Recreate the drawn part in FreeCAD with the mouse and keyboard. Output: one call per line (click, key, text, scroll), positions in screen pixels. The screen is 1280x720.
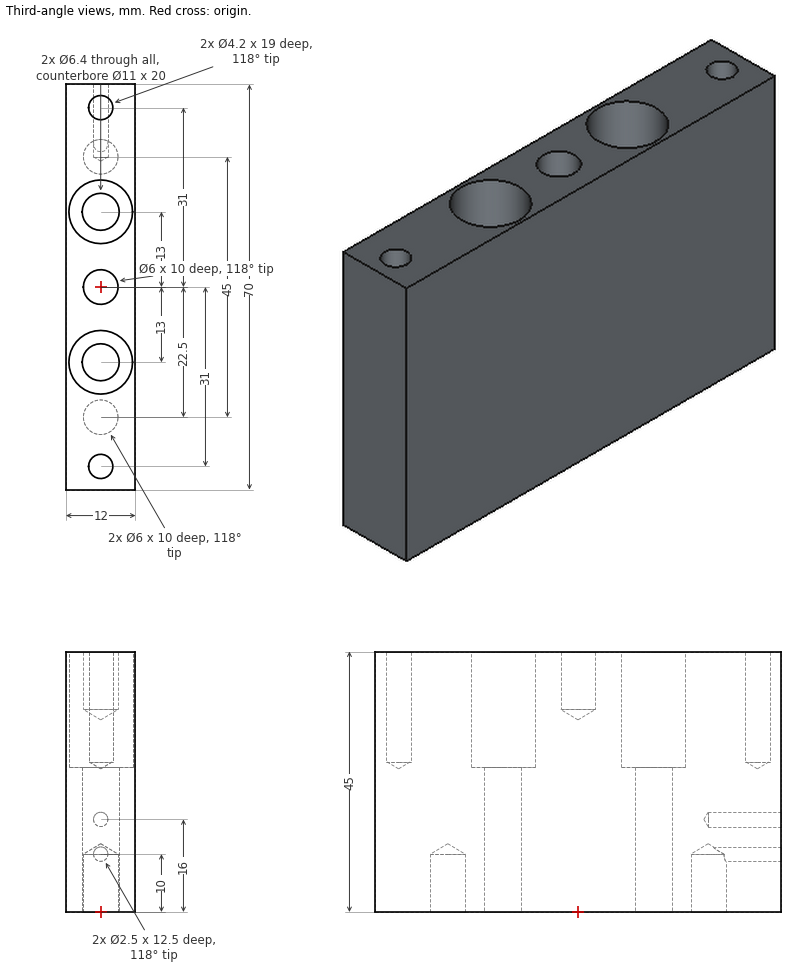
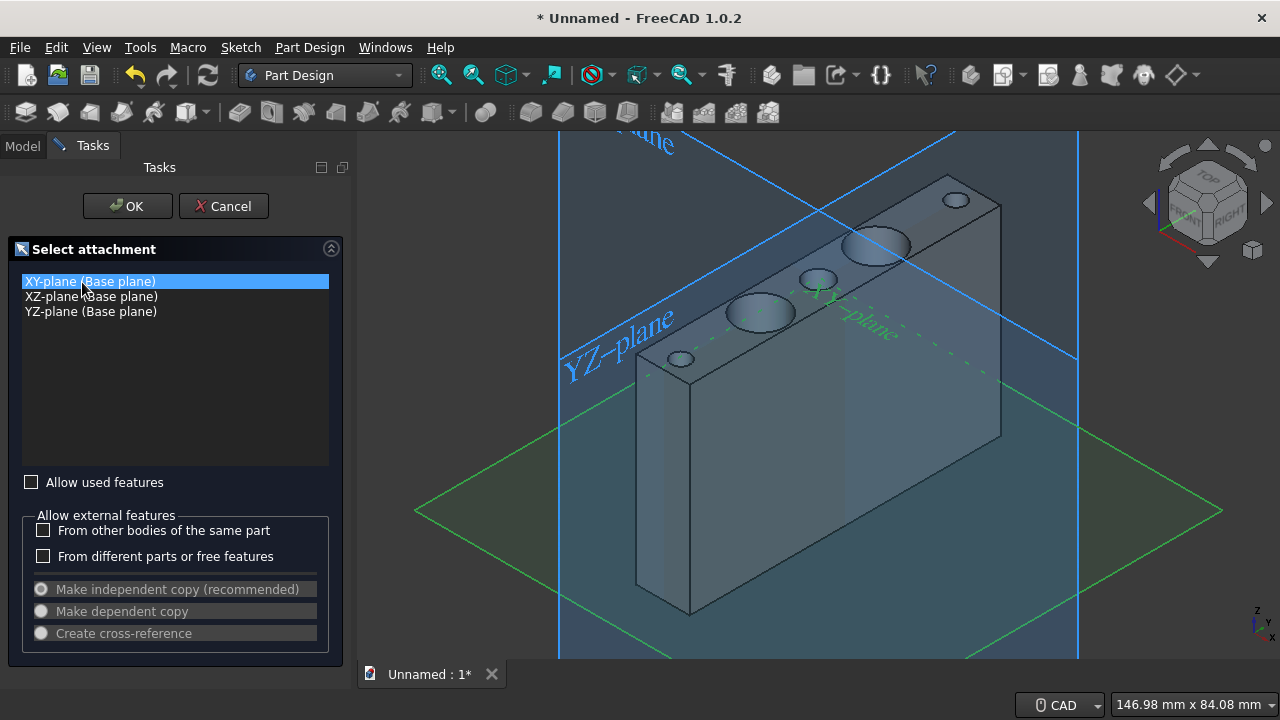
click(128, 206)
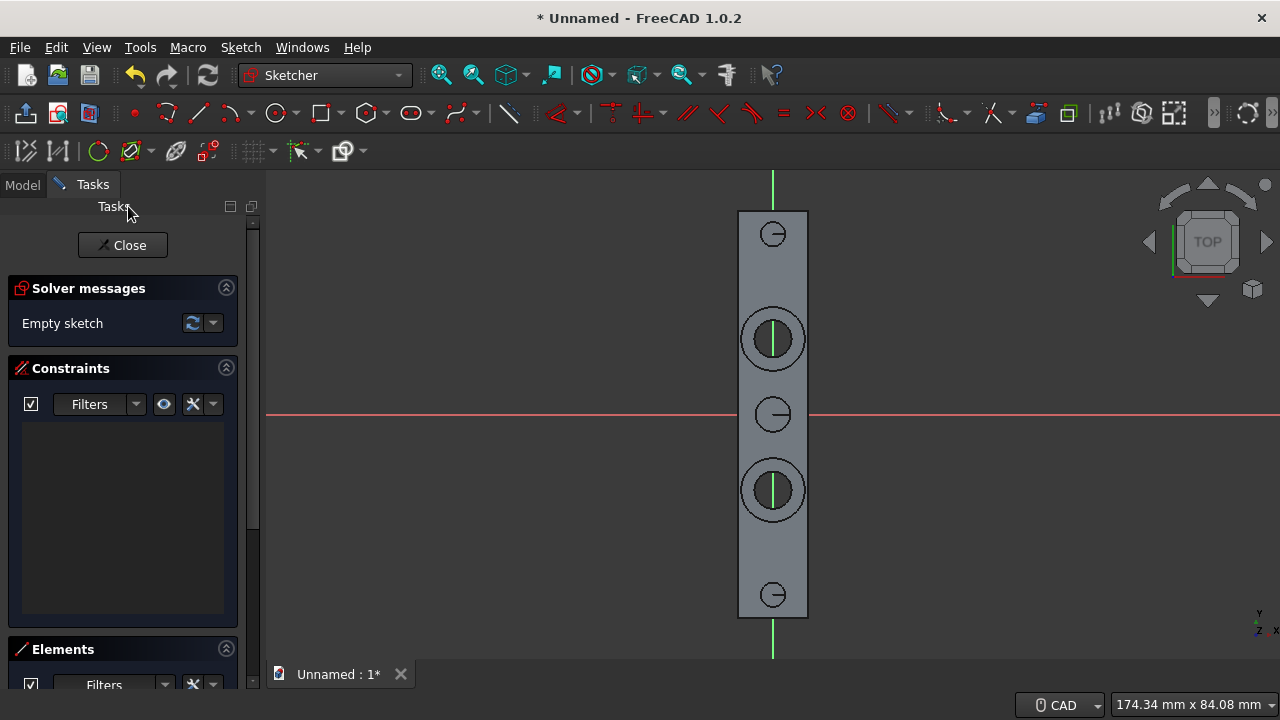
click(90, 114)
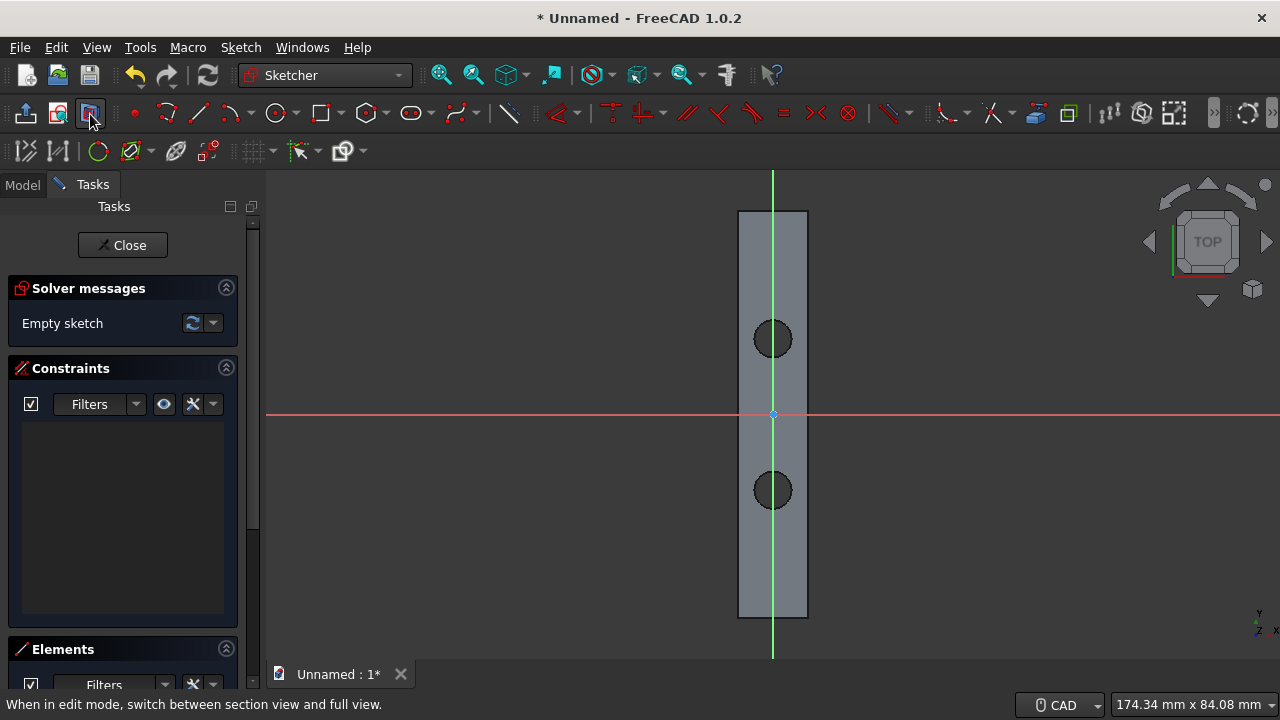
click(276, 114)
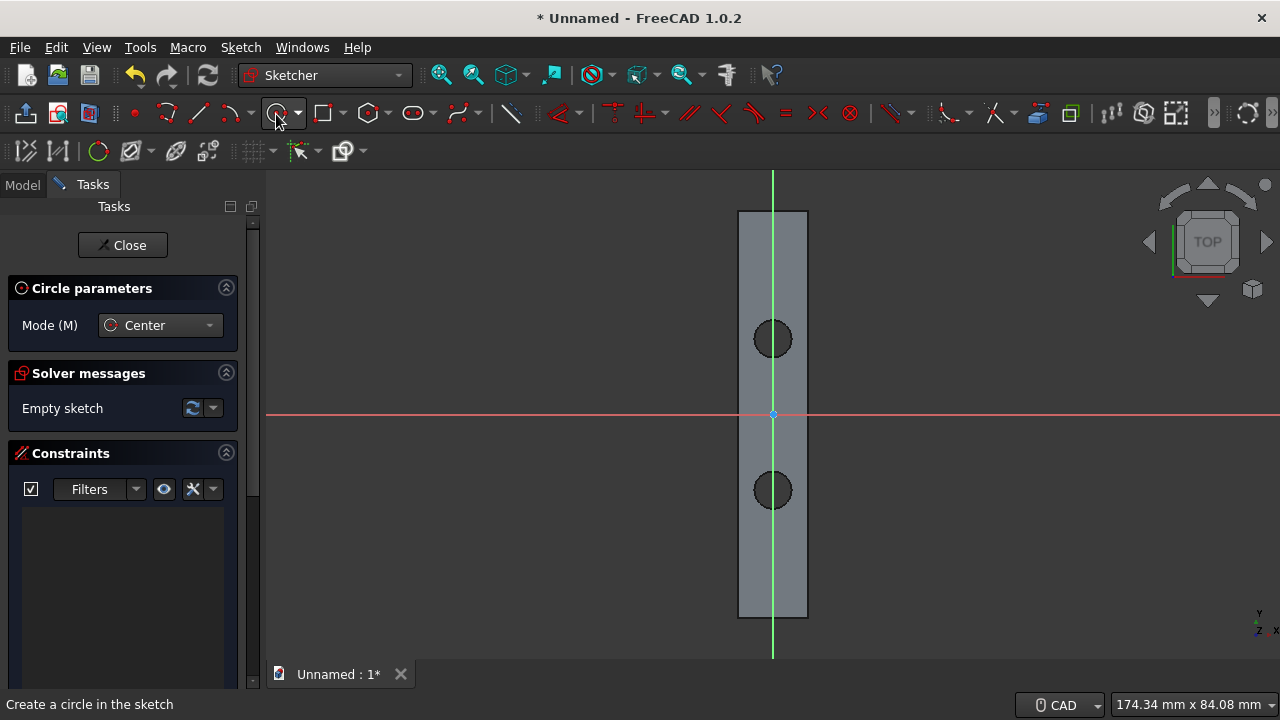
scroll(773, 545, up, 2)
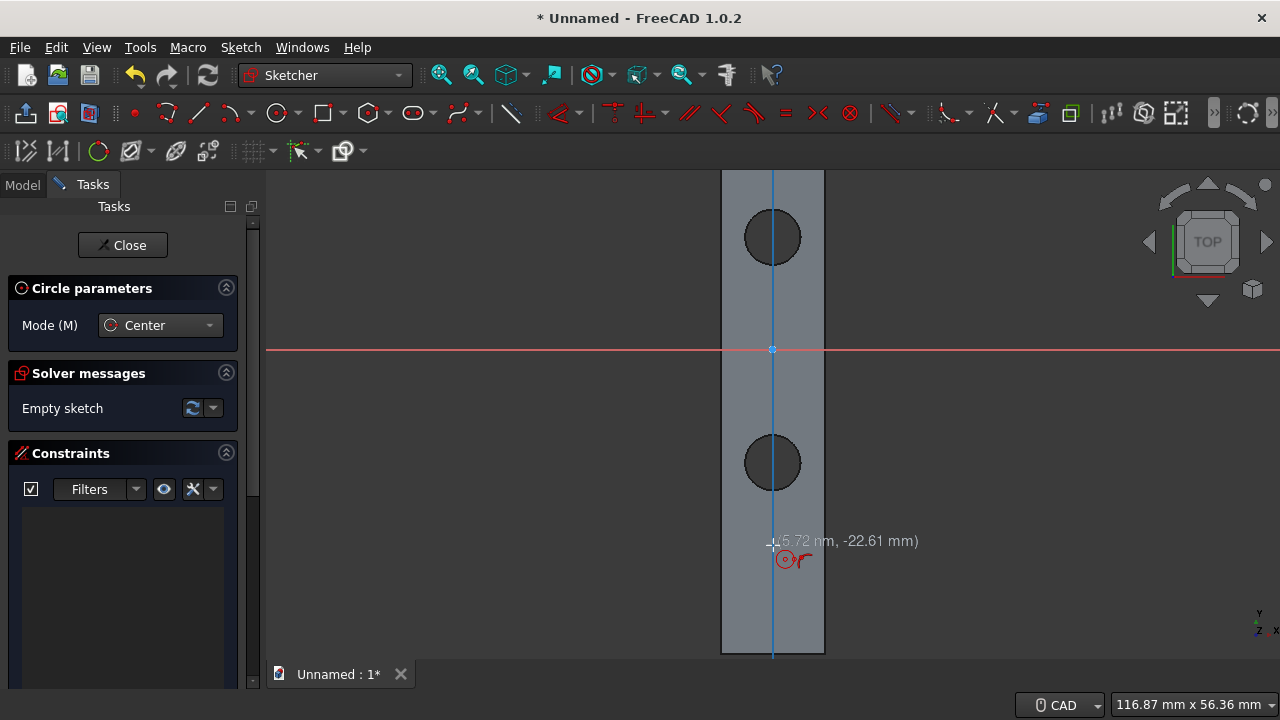
click(773, 545)
move(791, 527)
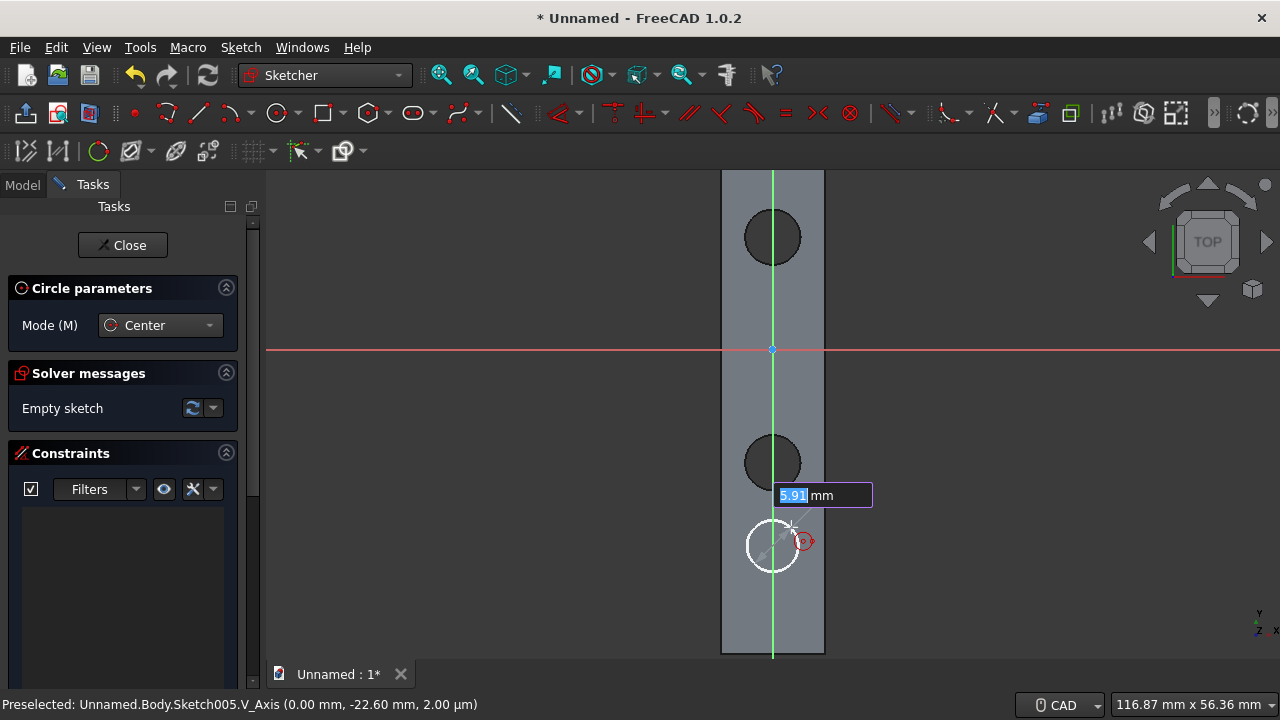
text(6)
key(Return)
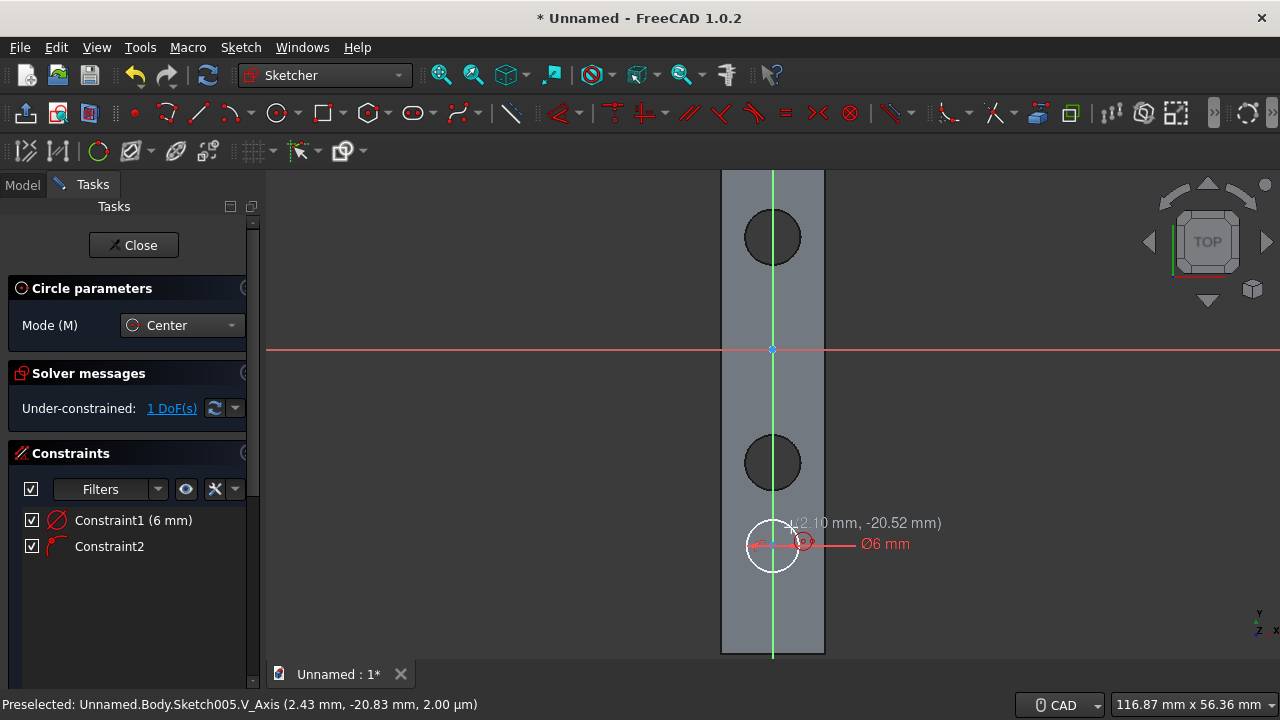
scroll(566, 546, down, 2)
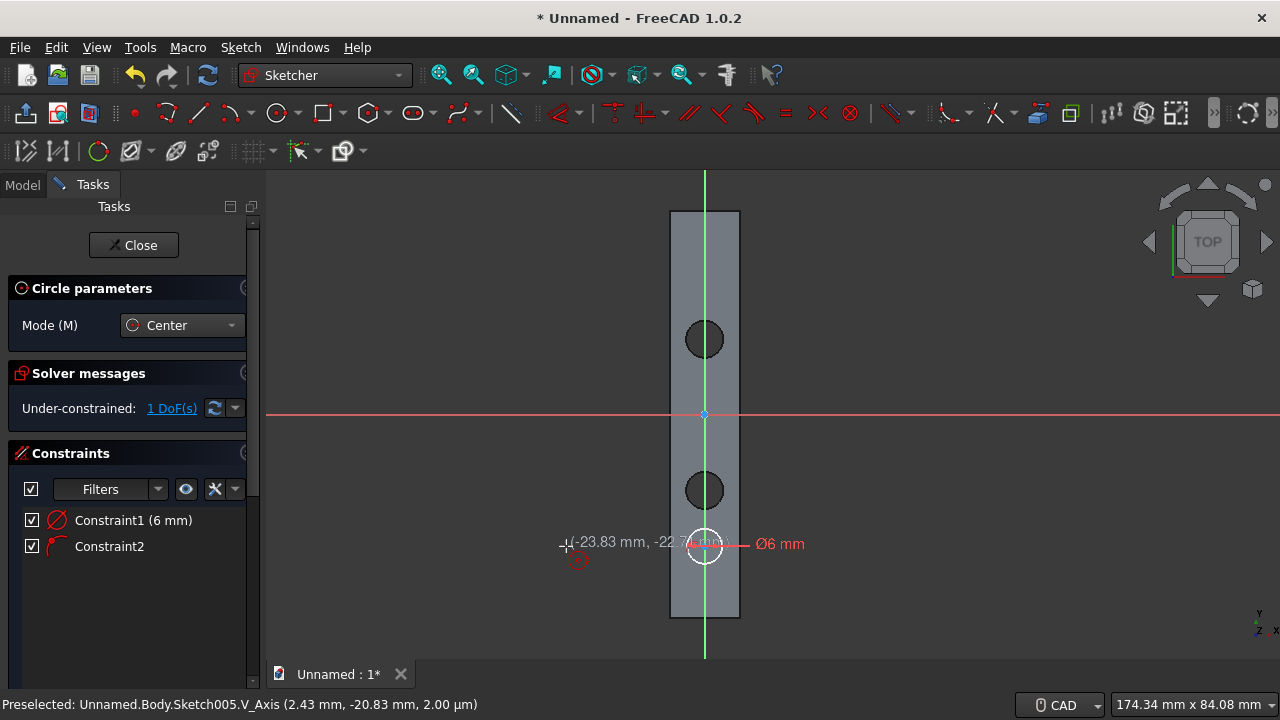
scroll(705, 284, up, 2)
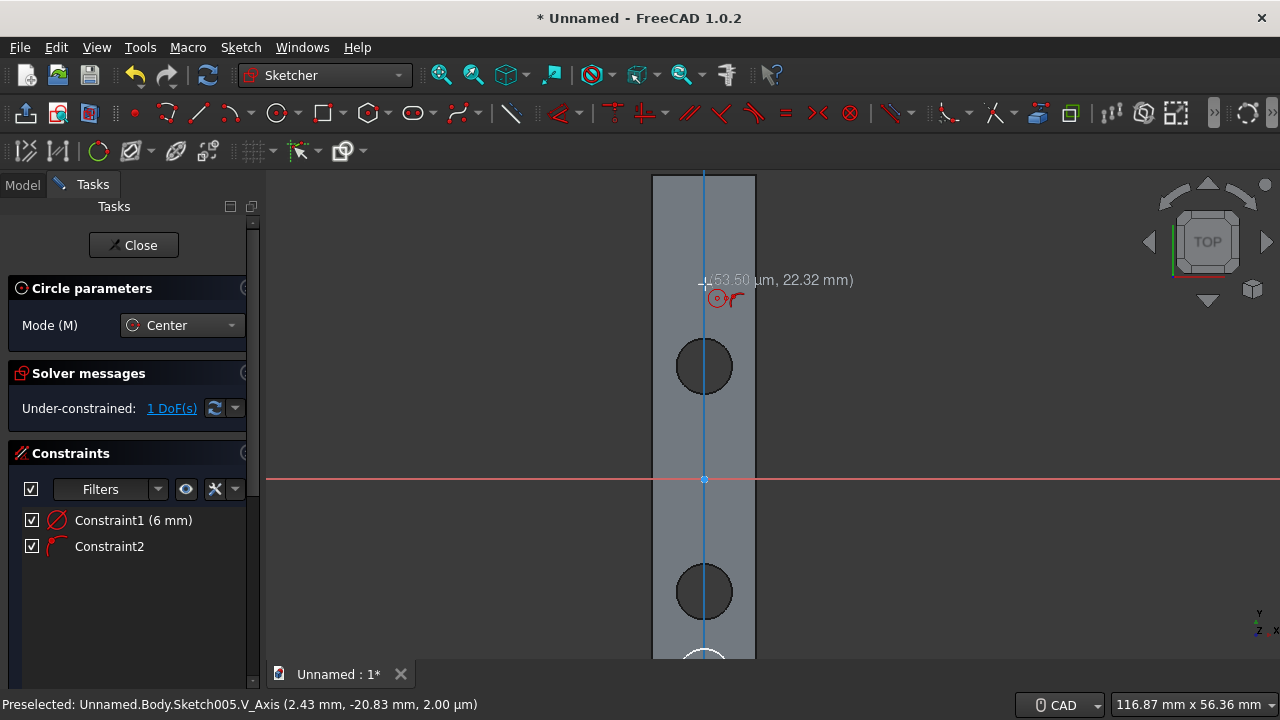
click(704, 284)
move(723, 265)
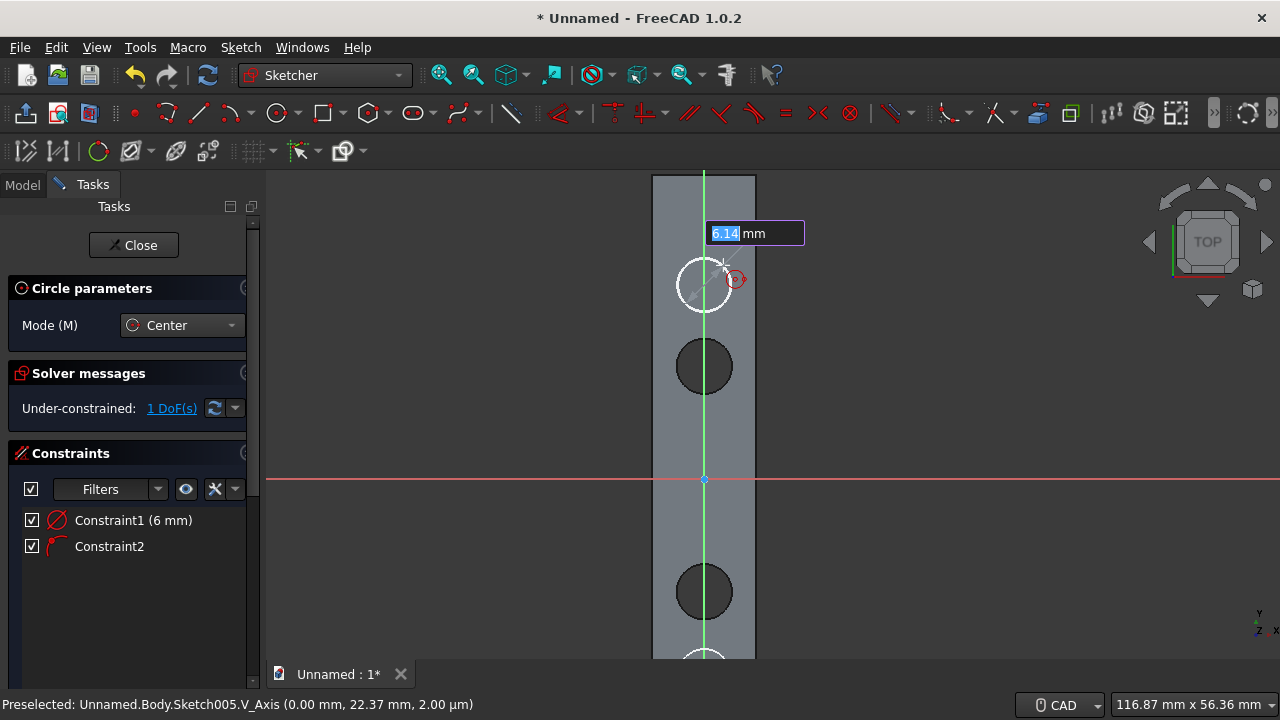
text(6)
key(Return)
key(Escape)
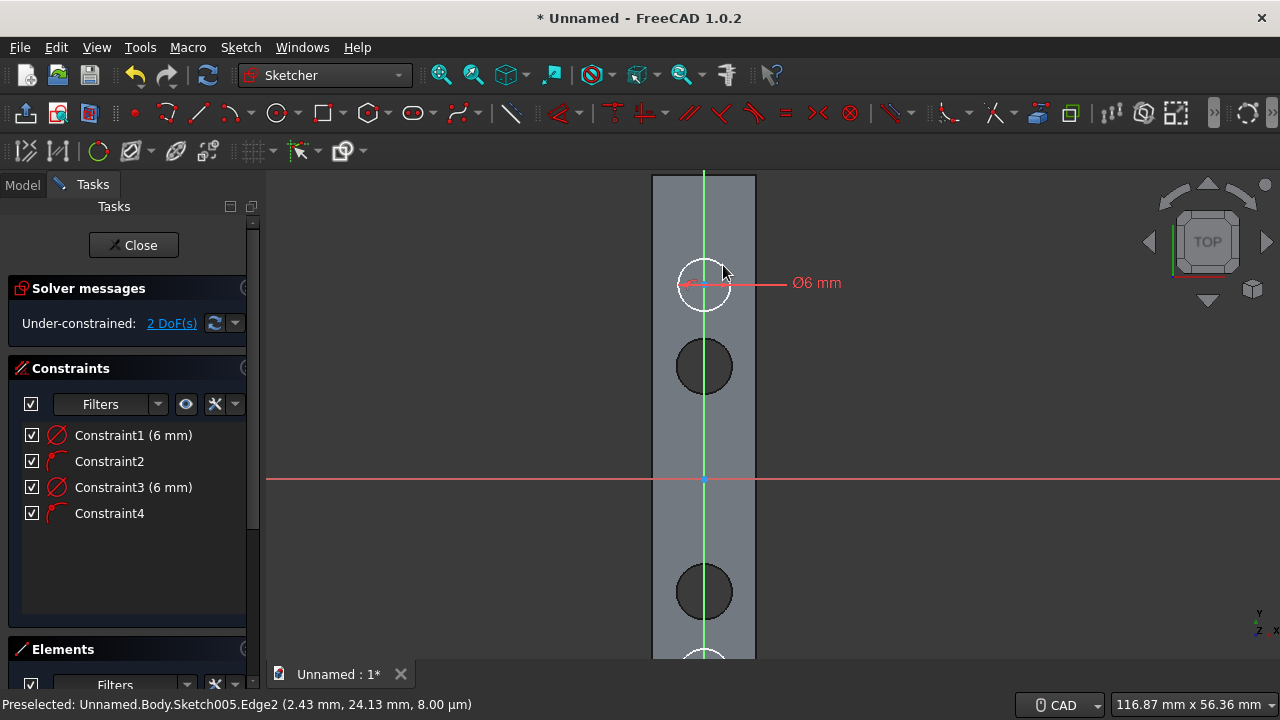
click(558, 114)